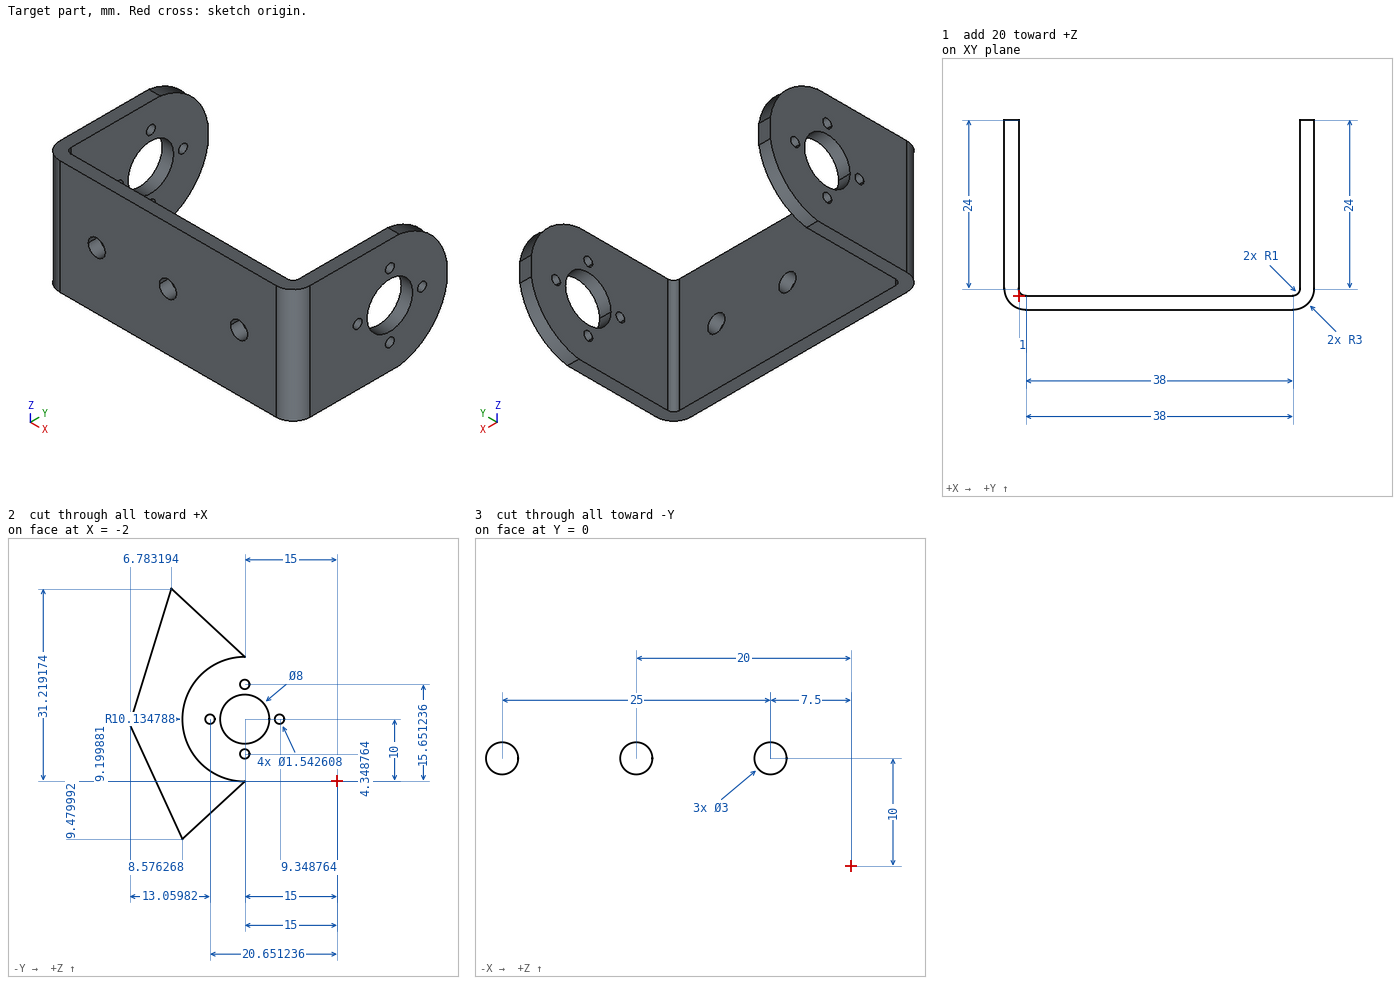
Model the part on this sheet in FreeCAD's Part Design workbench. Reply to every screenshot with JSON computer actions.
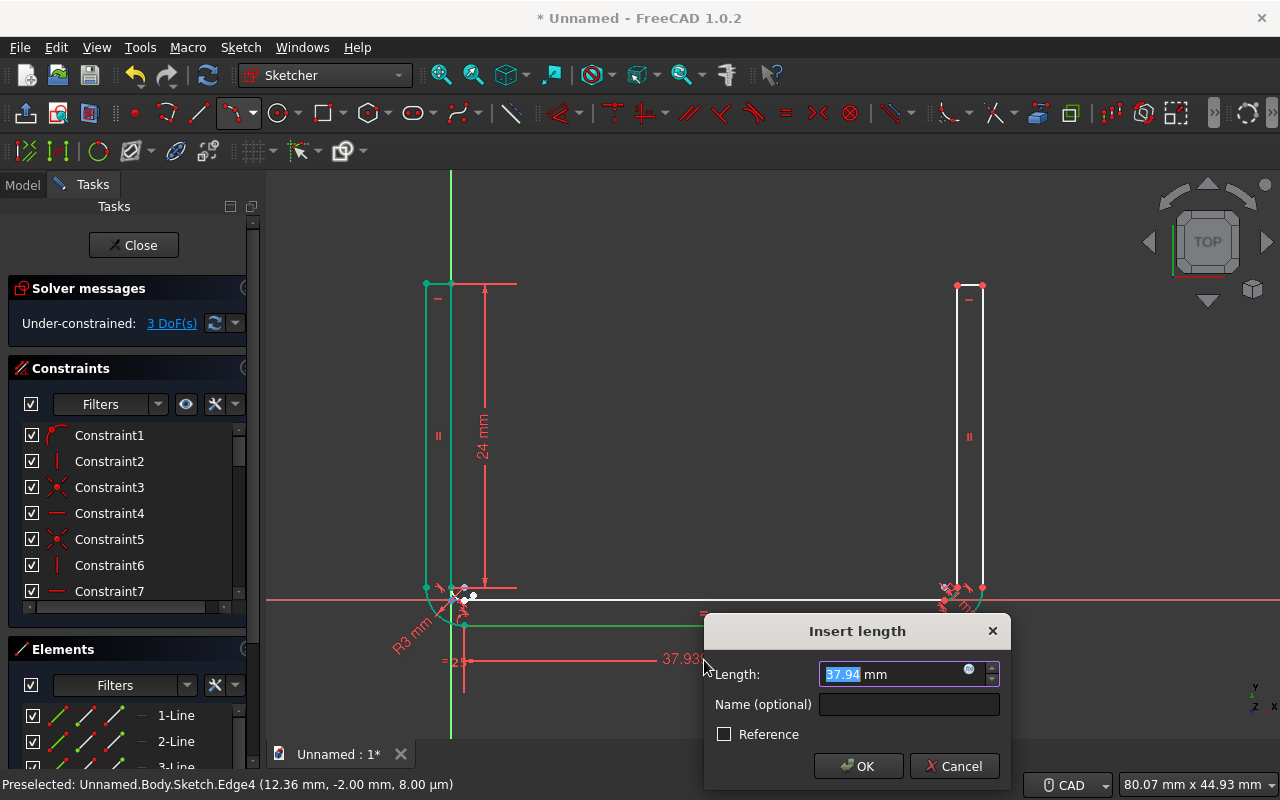
{"action": "type", "text": "38"}
{"action": "key", "text": "Return"}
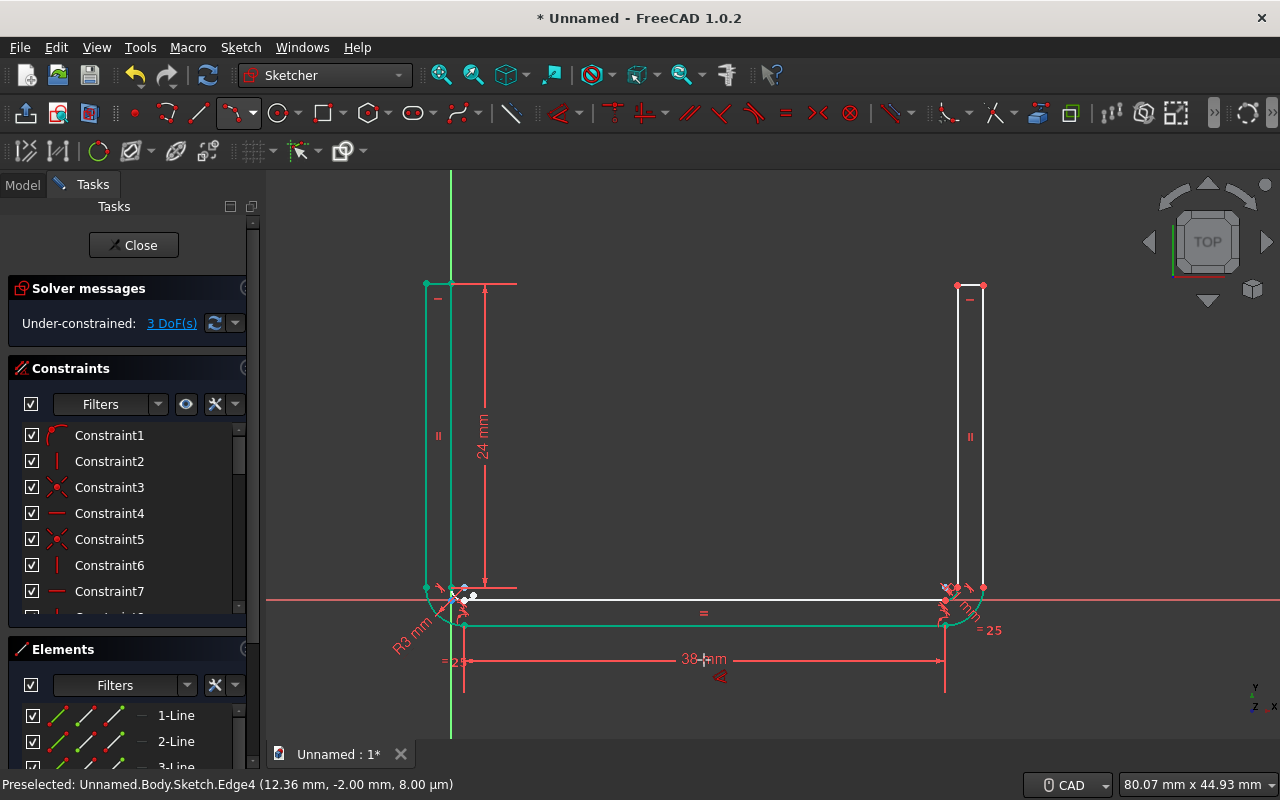
{"action": "left_click", "coordinate": [983, 497]}
{"action": "left_click", "coordinate": [1017, 436]}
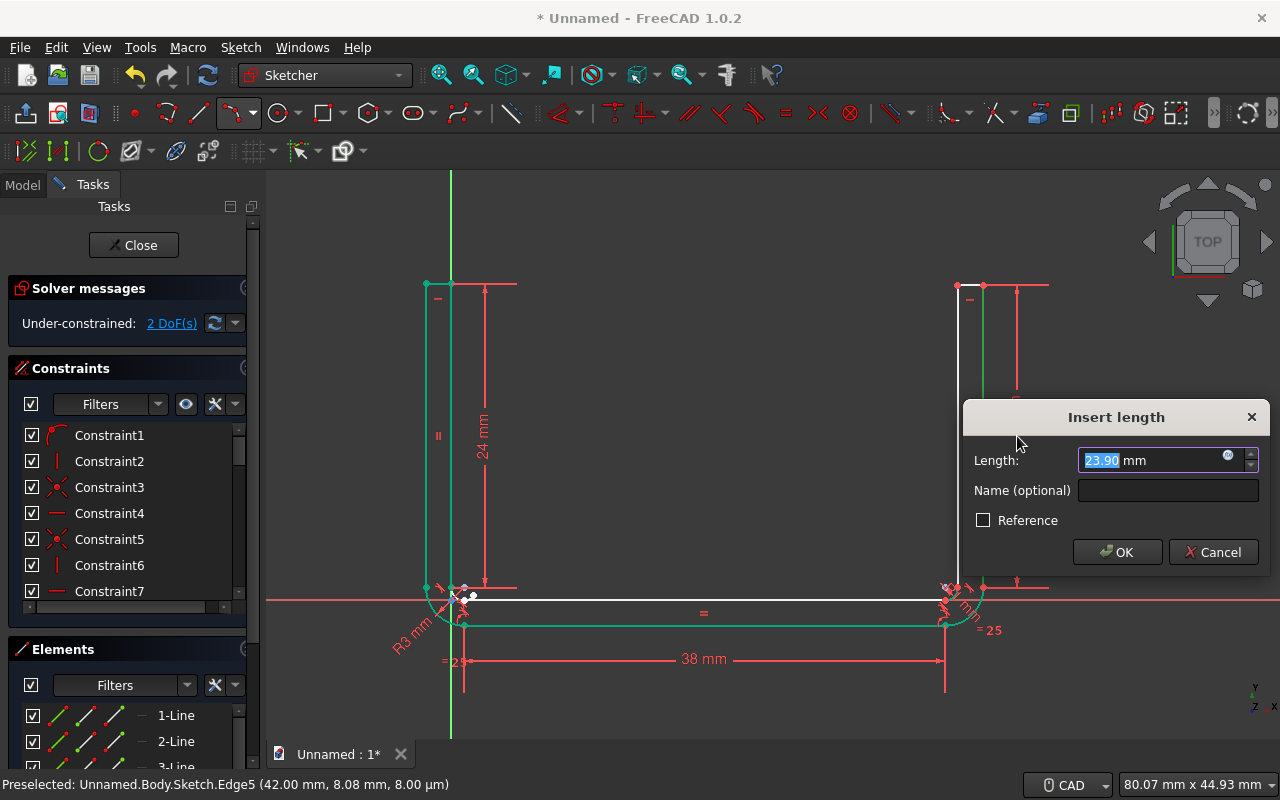
{"action": "type", "text": "24"}
{"action": "key", "text": "Return"}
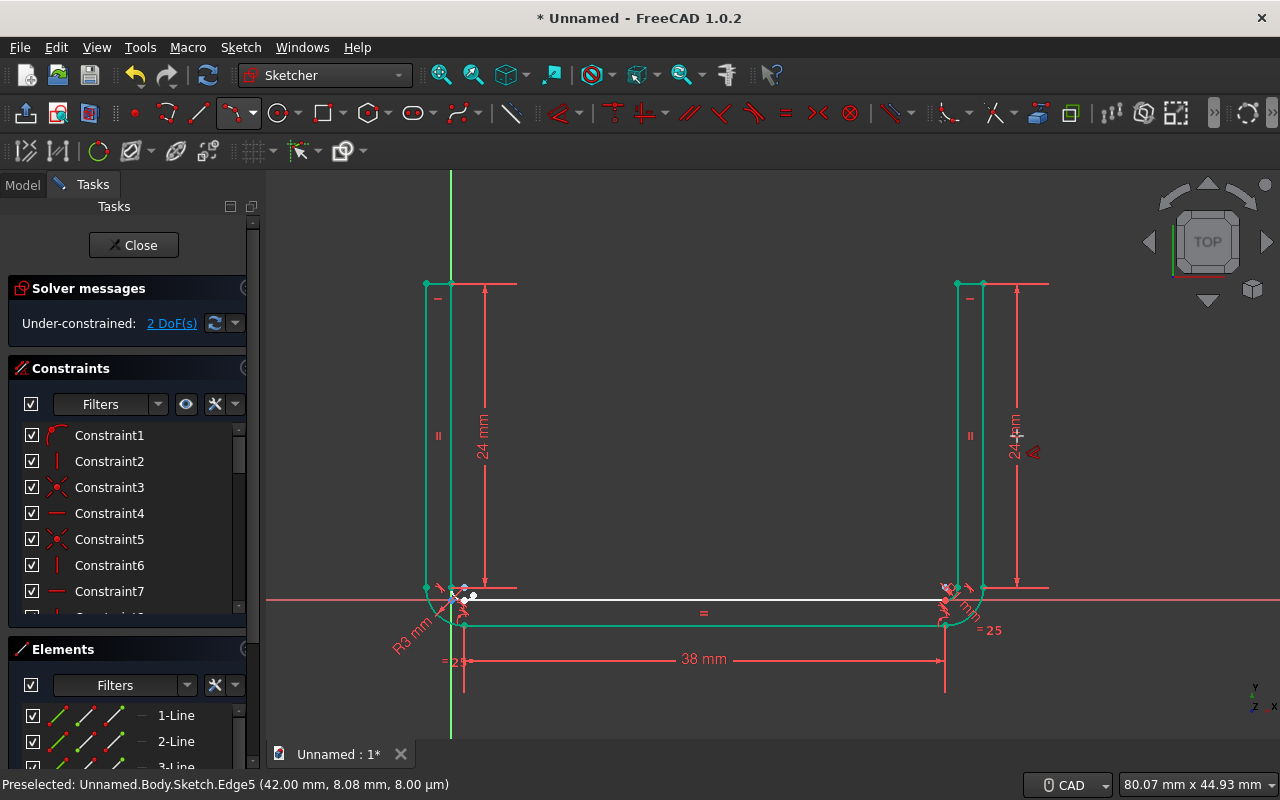
{"action": "left_click", "coordinate": [801, 600]}
{"action": "left_click", "coordinate": [705, 566]}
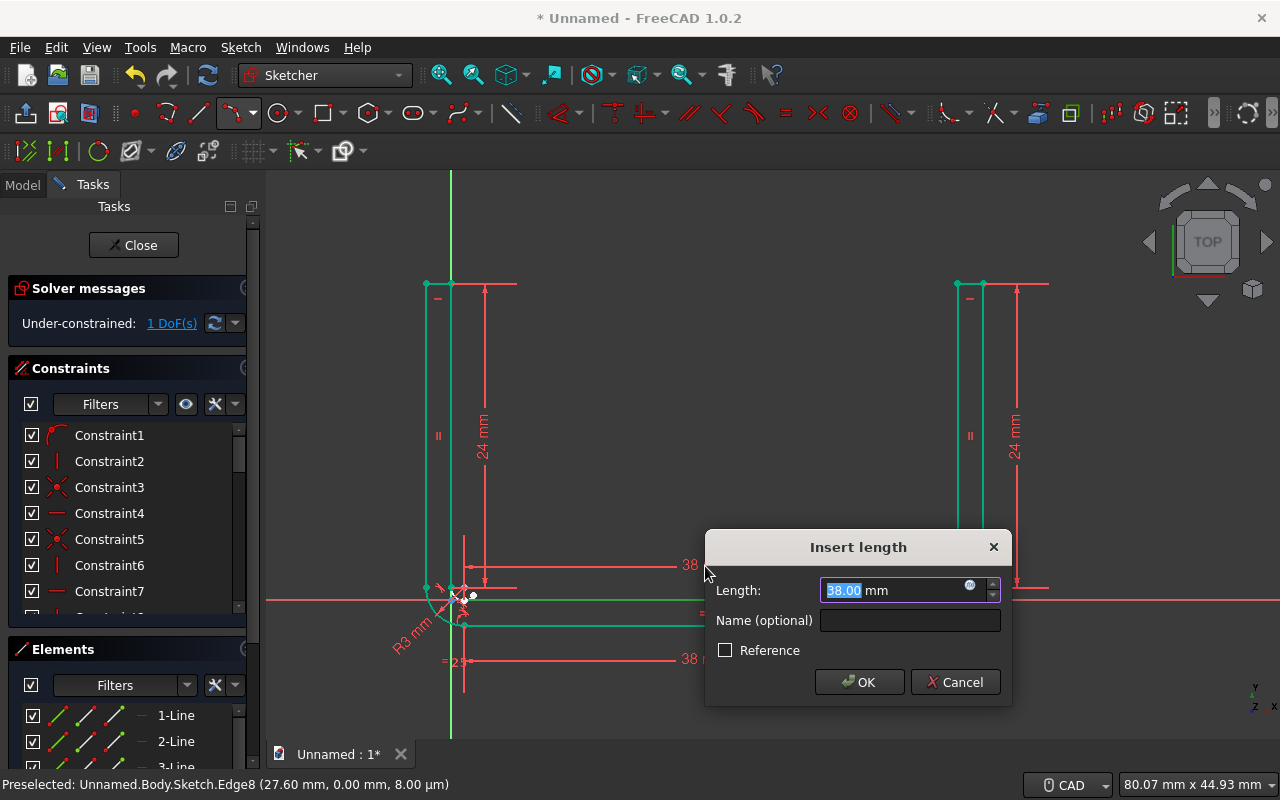
{"action": "type", "text": "38"}
{"action": "key", "text": "Return"}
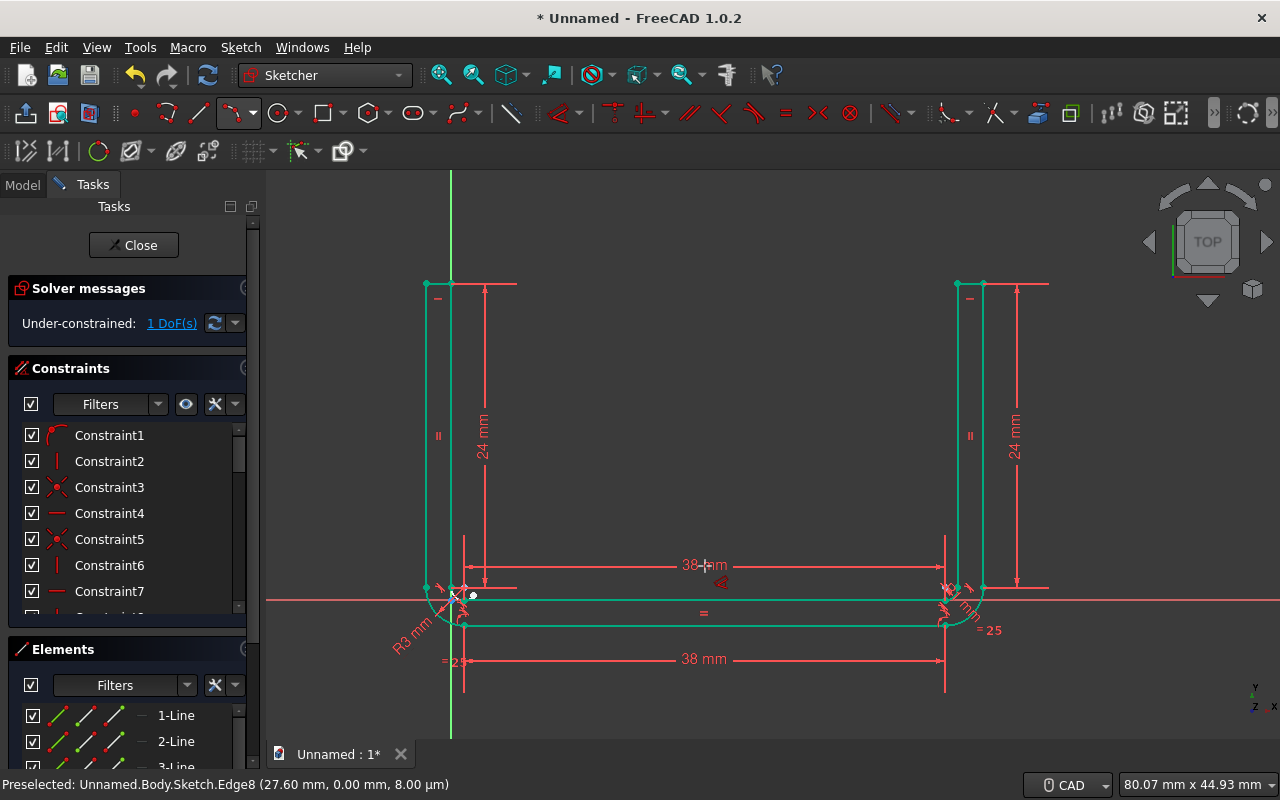
{"action": "scroll", "coordinate": [474, 596], "scroll_direction": "up", "scroll_amount": 6}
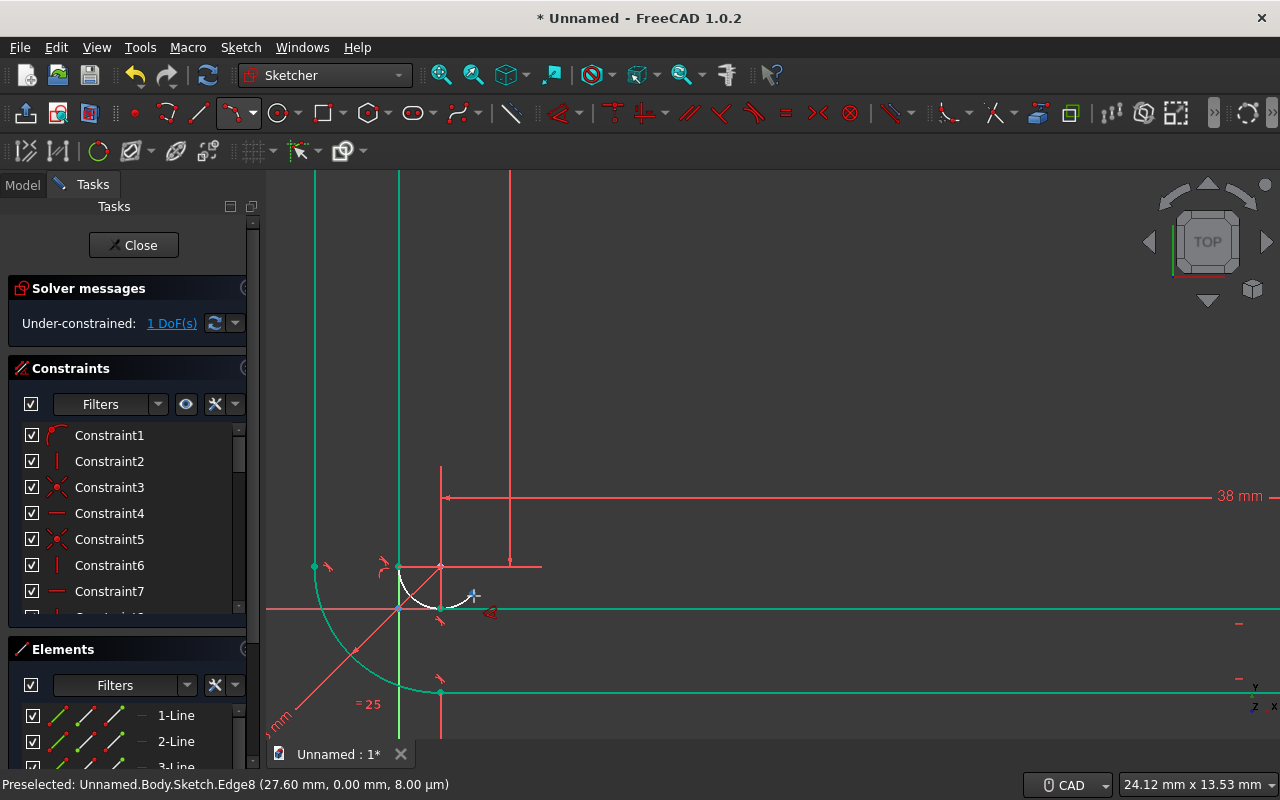
{"action": "left_click", "coordinate": [473, 594]}
{"action": "left_click", "coordinate": [436, 643]}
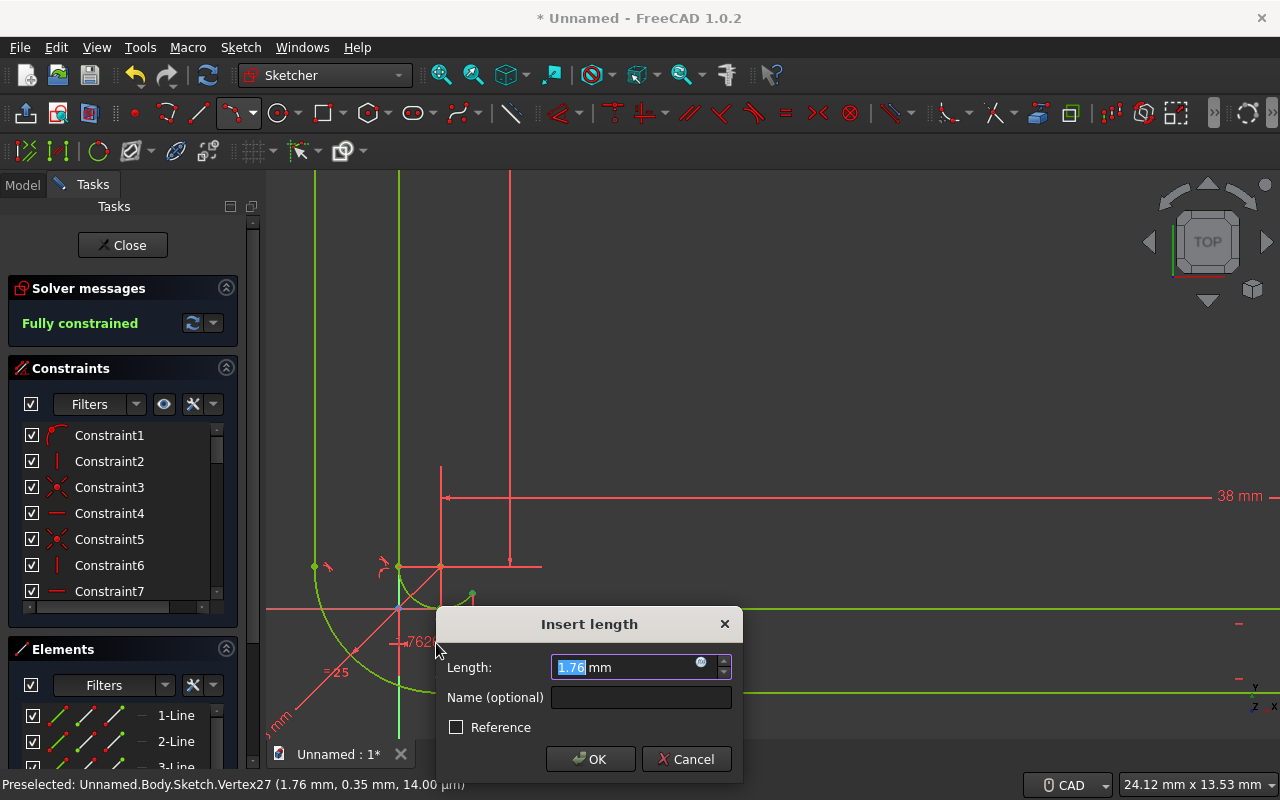
{"action": "type", "text": "1"}
{"action": "key", "text": "Return"}
{"action": "key", "text": "Escape"}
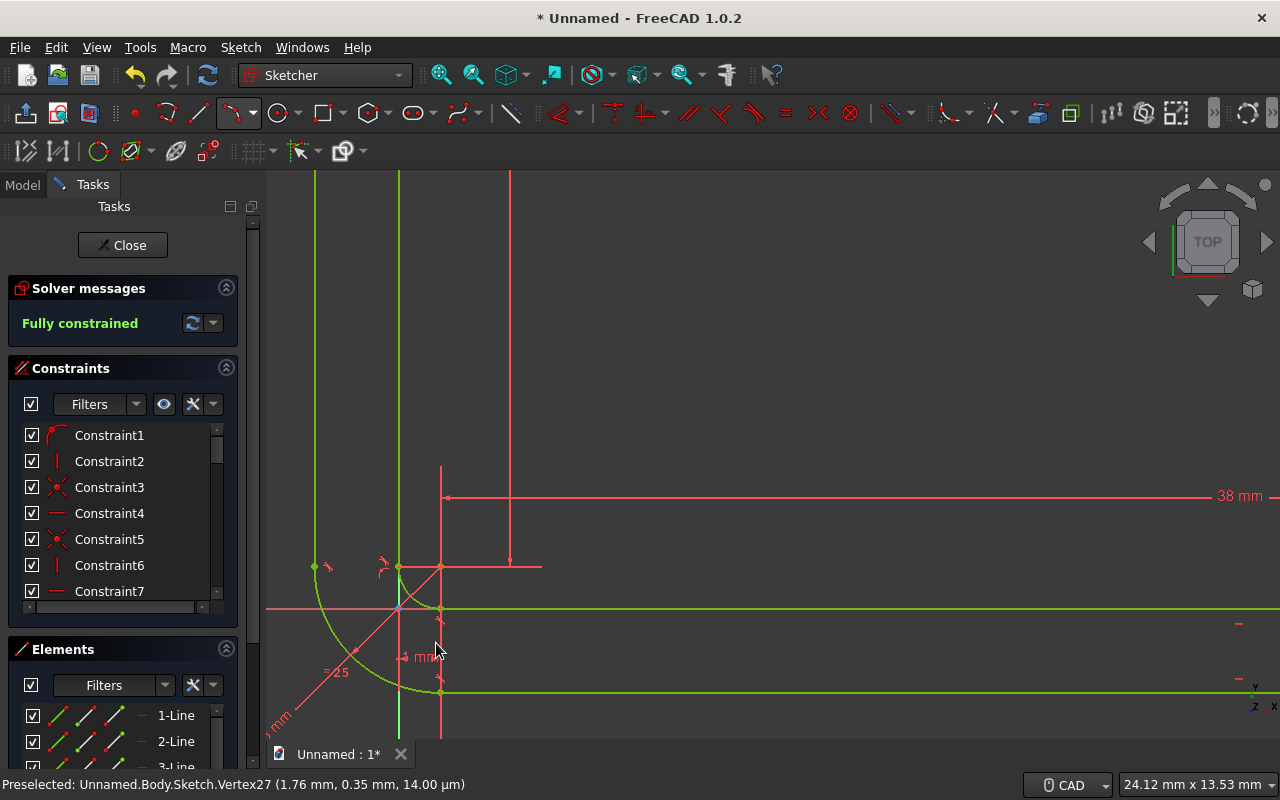
{"action": "left_click", "coordinate": [123, 245]}